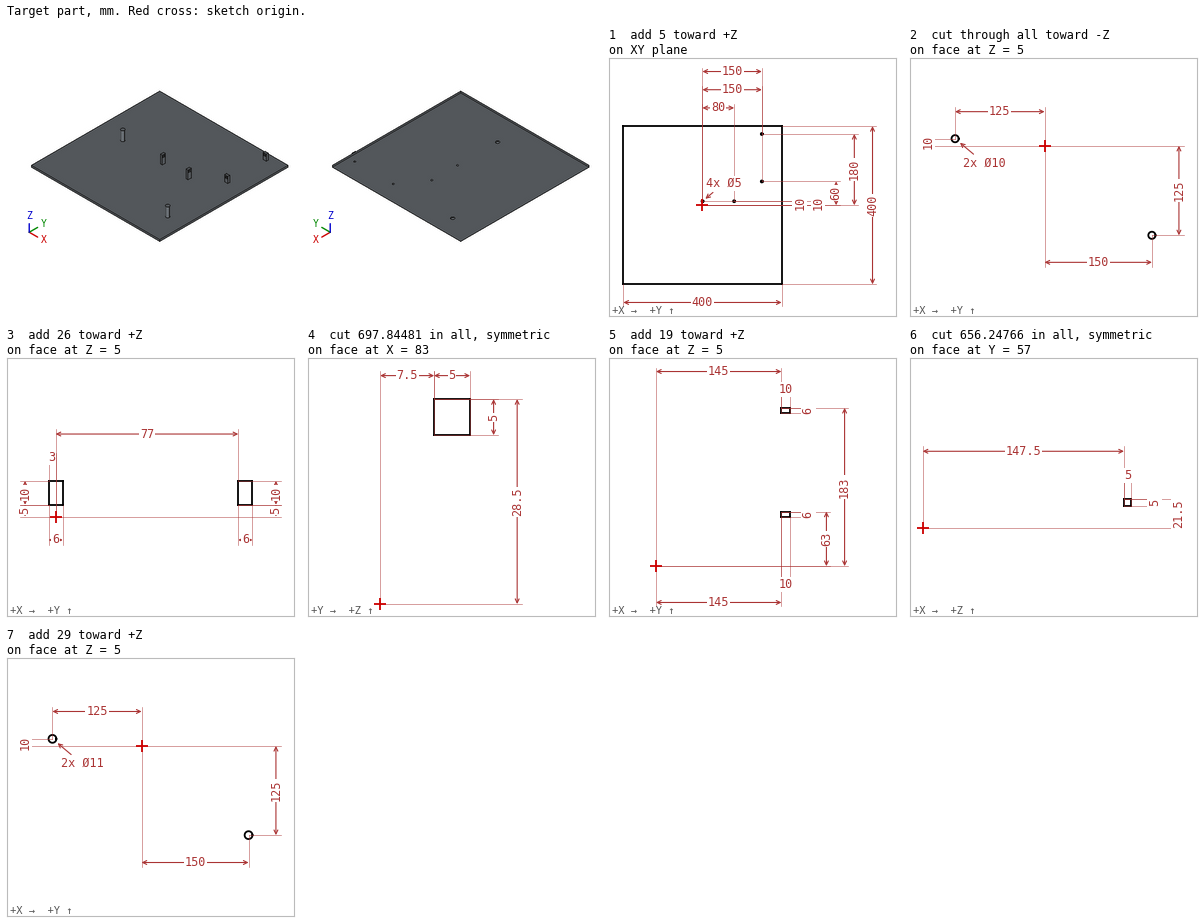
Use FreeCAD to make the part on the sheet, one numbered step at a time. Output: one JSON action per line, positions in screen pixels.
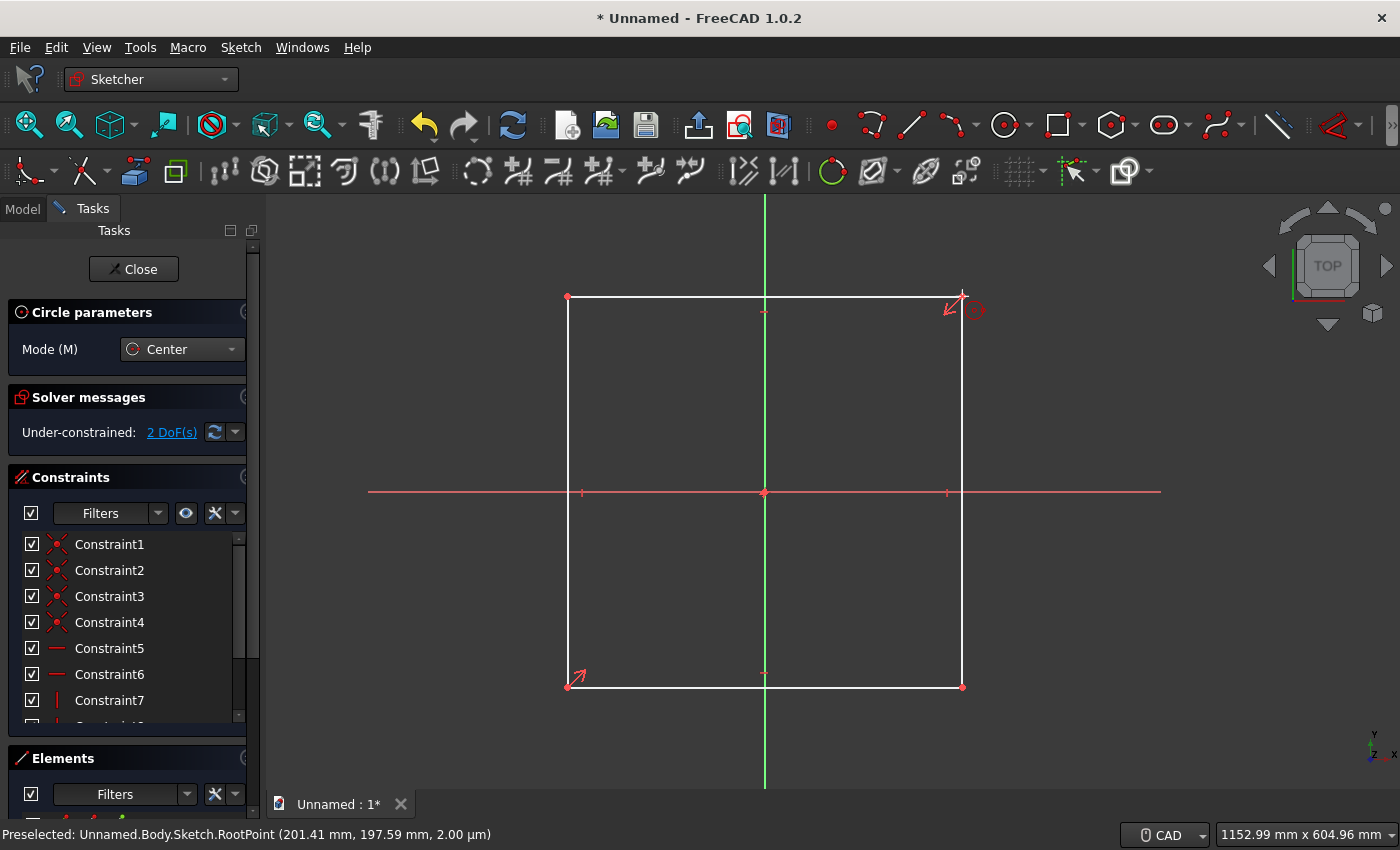
{"action": "scroll", "coordinate": [765, 483], "scroll_direction": "up", "scroll_amount": 12}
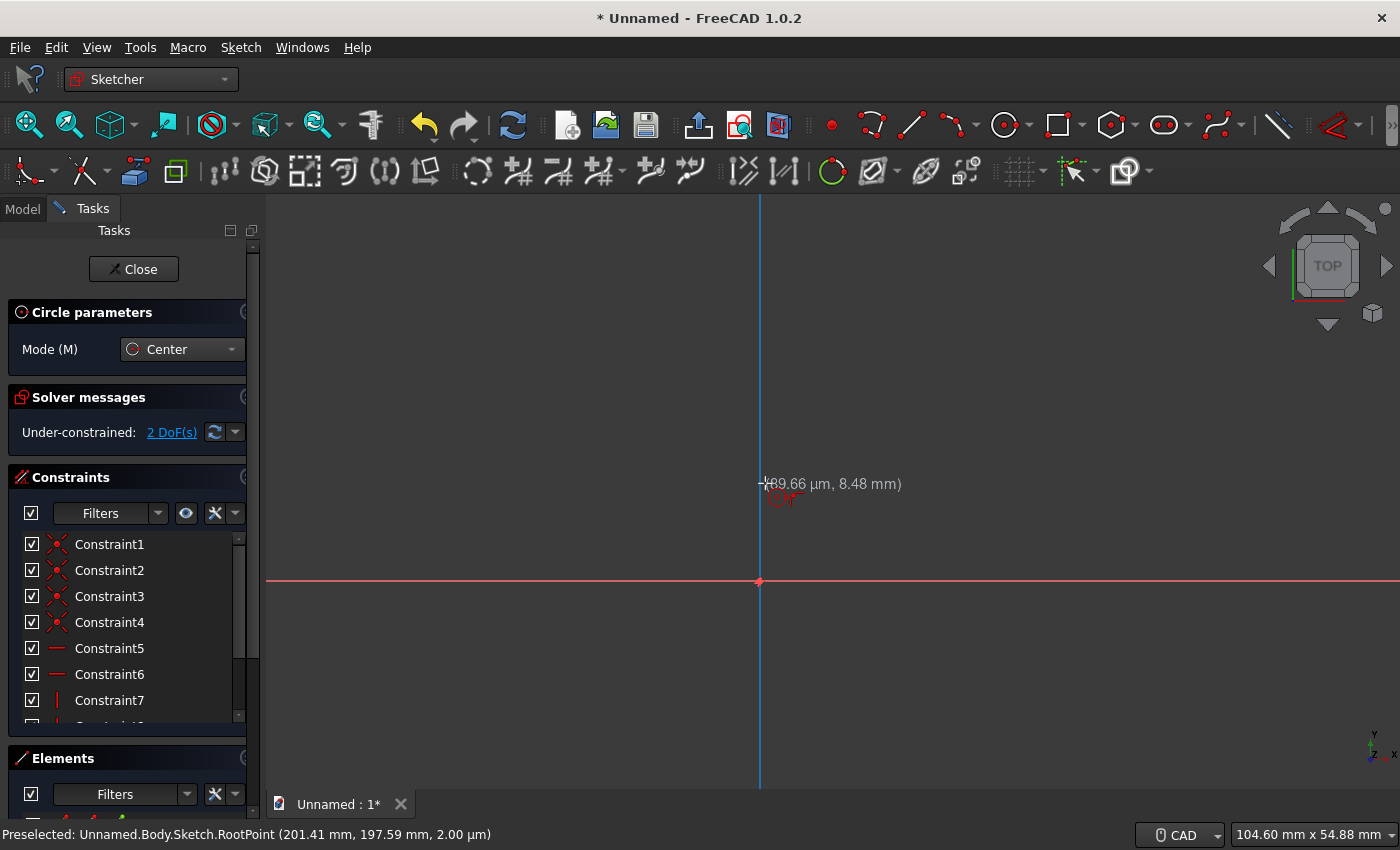
{"action": "scroll", "coordinate": [765, 483], "scroll_direction": "down", "scroll_amount": 12}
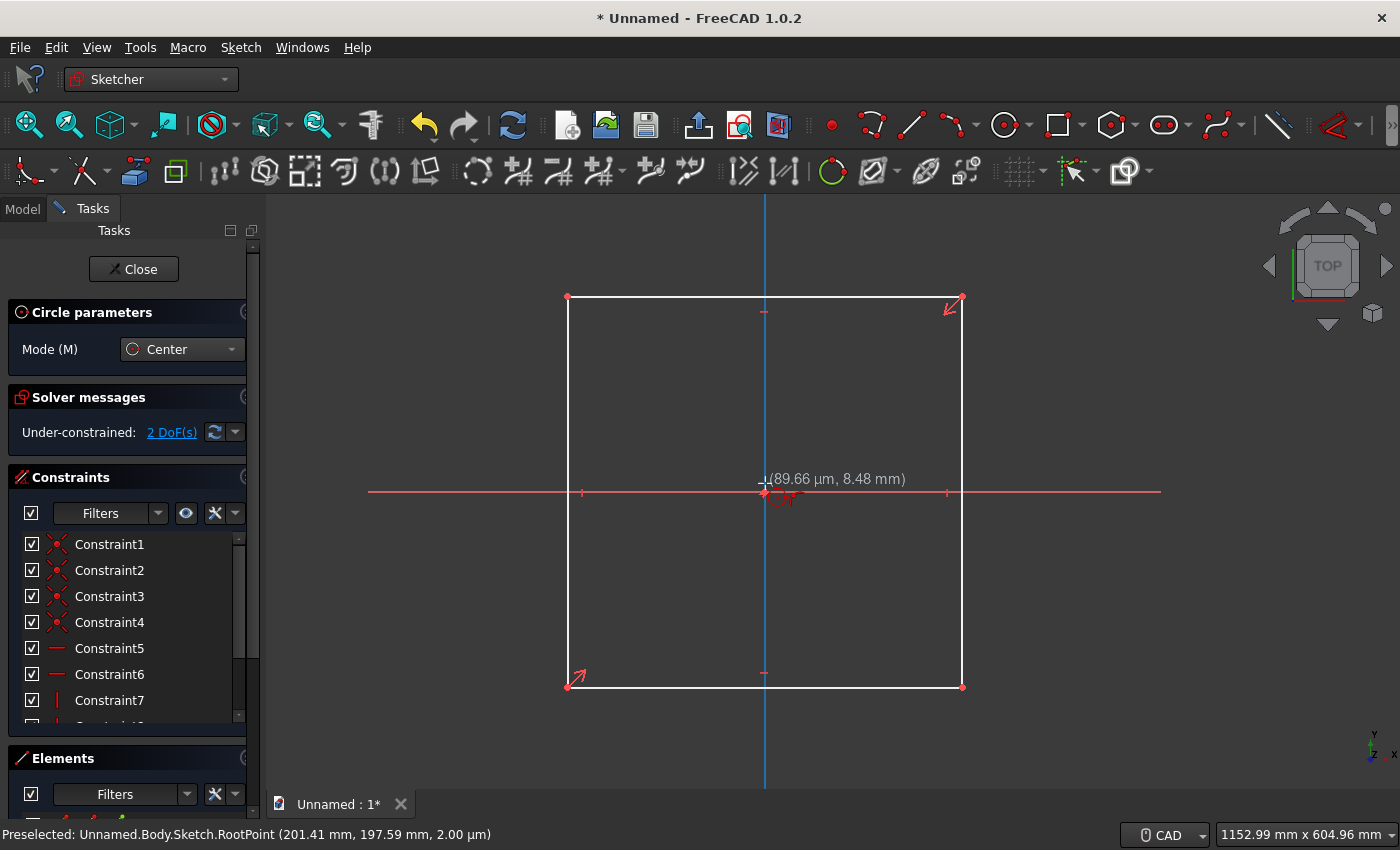
{"action": "scroll", "coordinate": [765, 483], "scroll_direction": "up", "scroll_amount": 3}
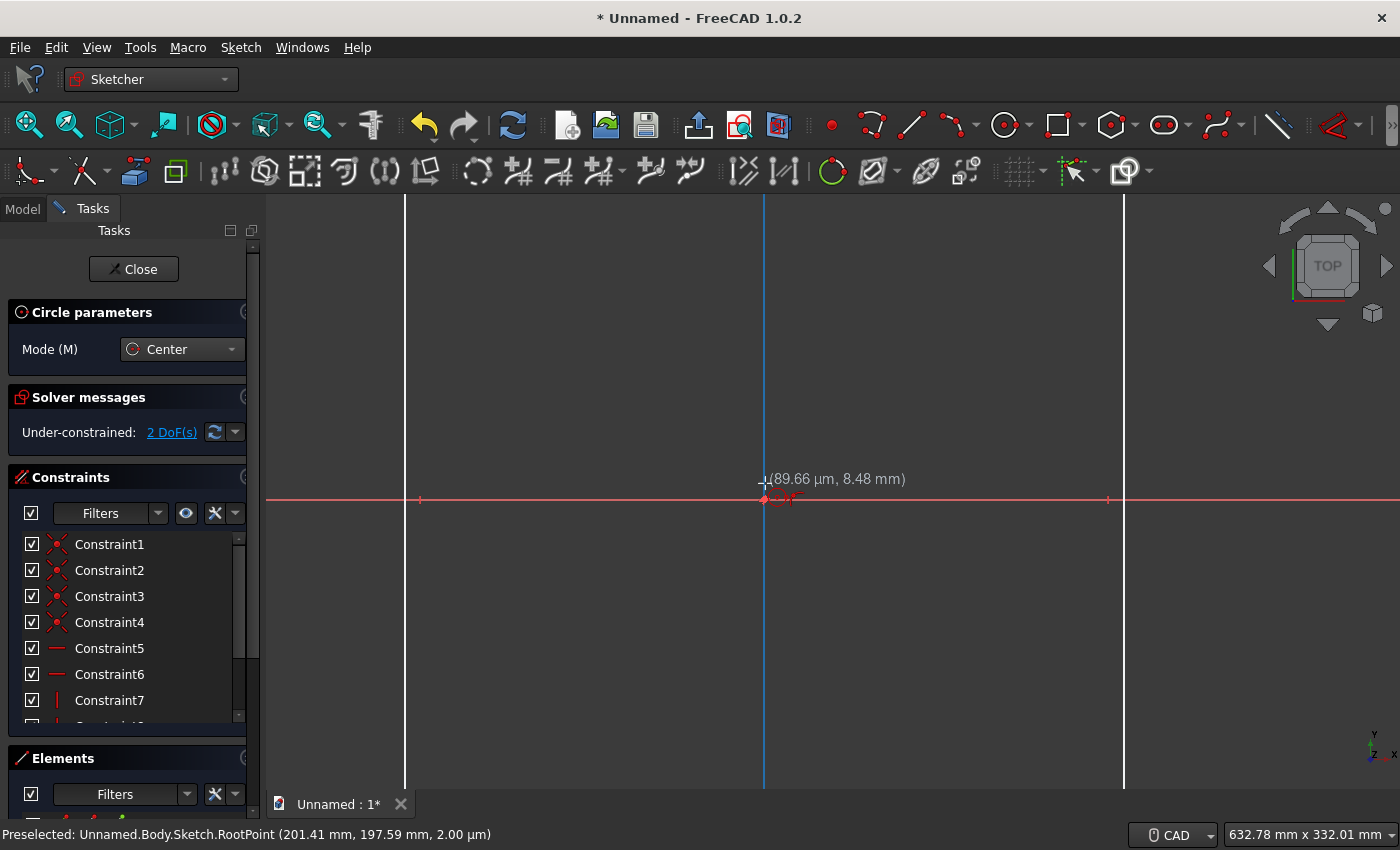
{"action": "left_click", "coordinate": [764, 482]}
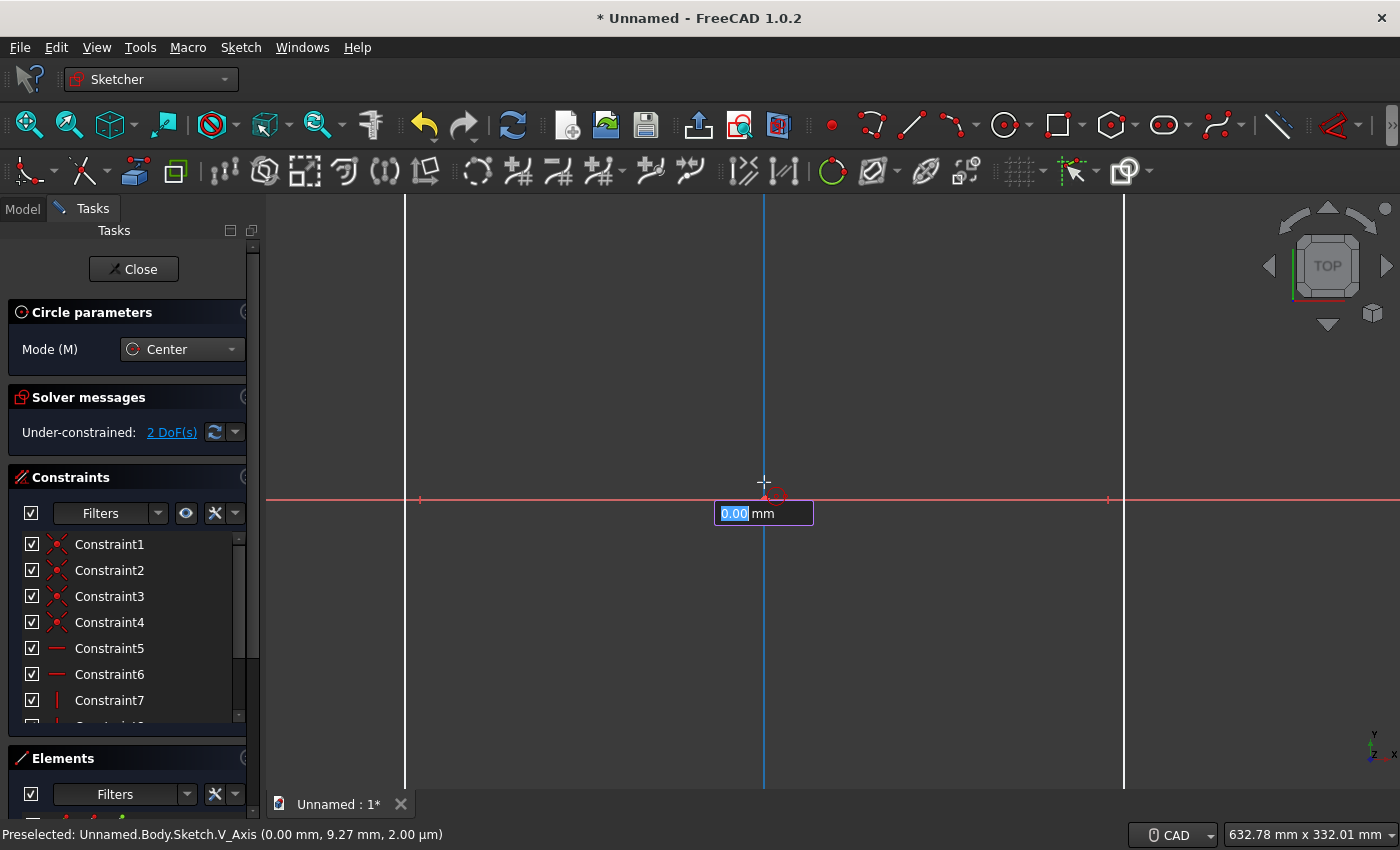
{"action": "scroll", "coordinate": [769, 480], "scroll_direction": "up", "scroll_amount": 7}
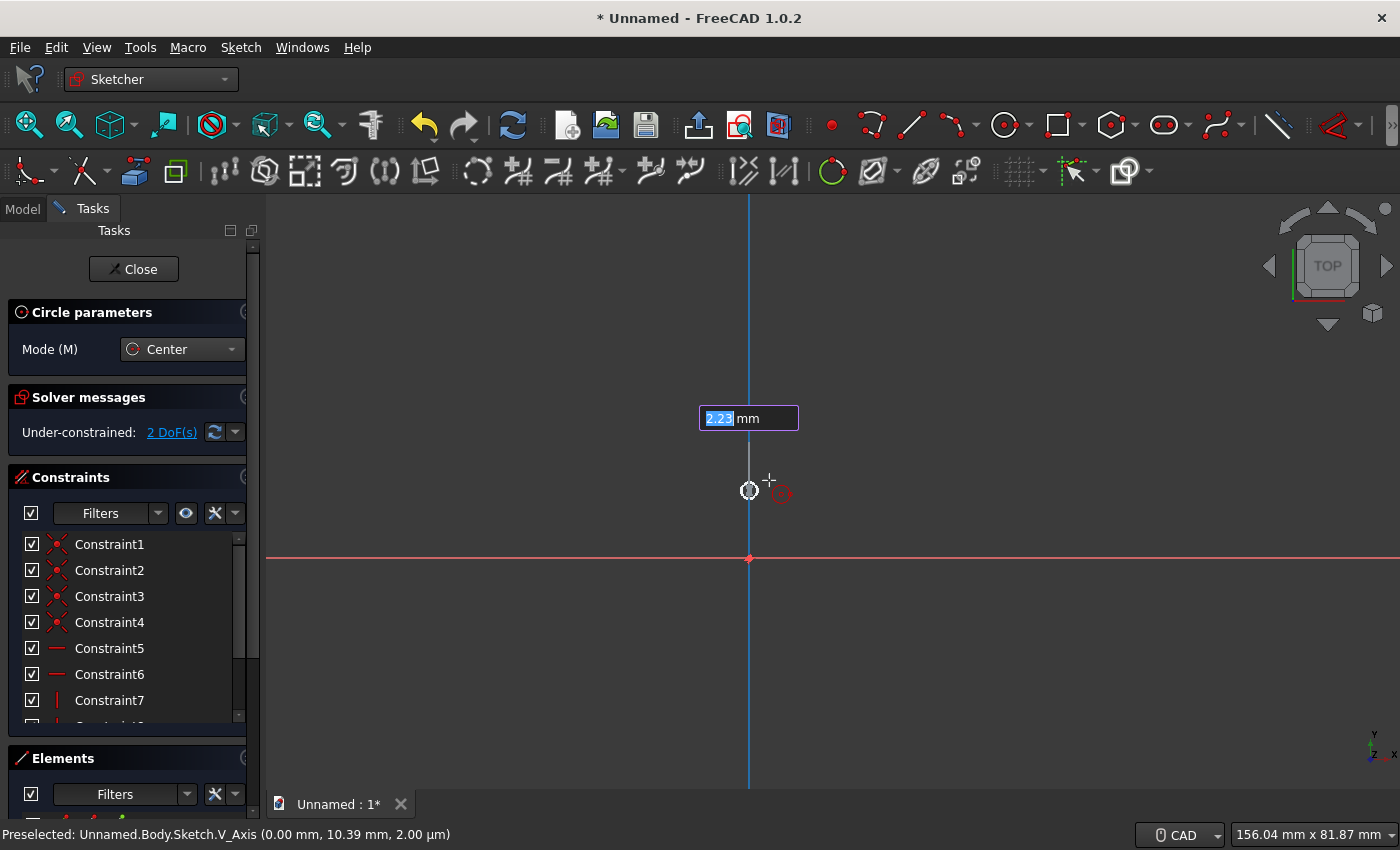
{"action": "left_click", "coordinate": [766, 479]}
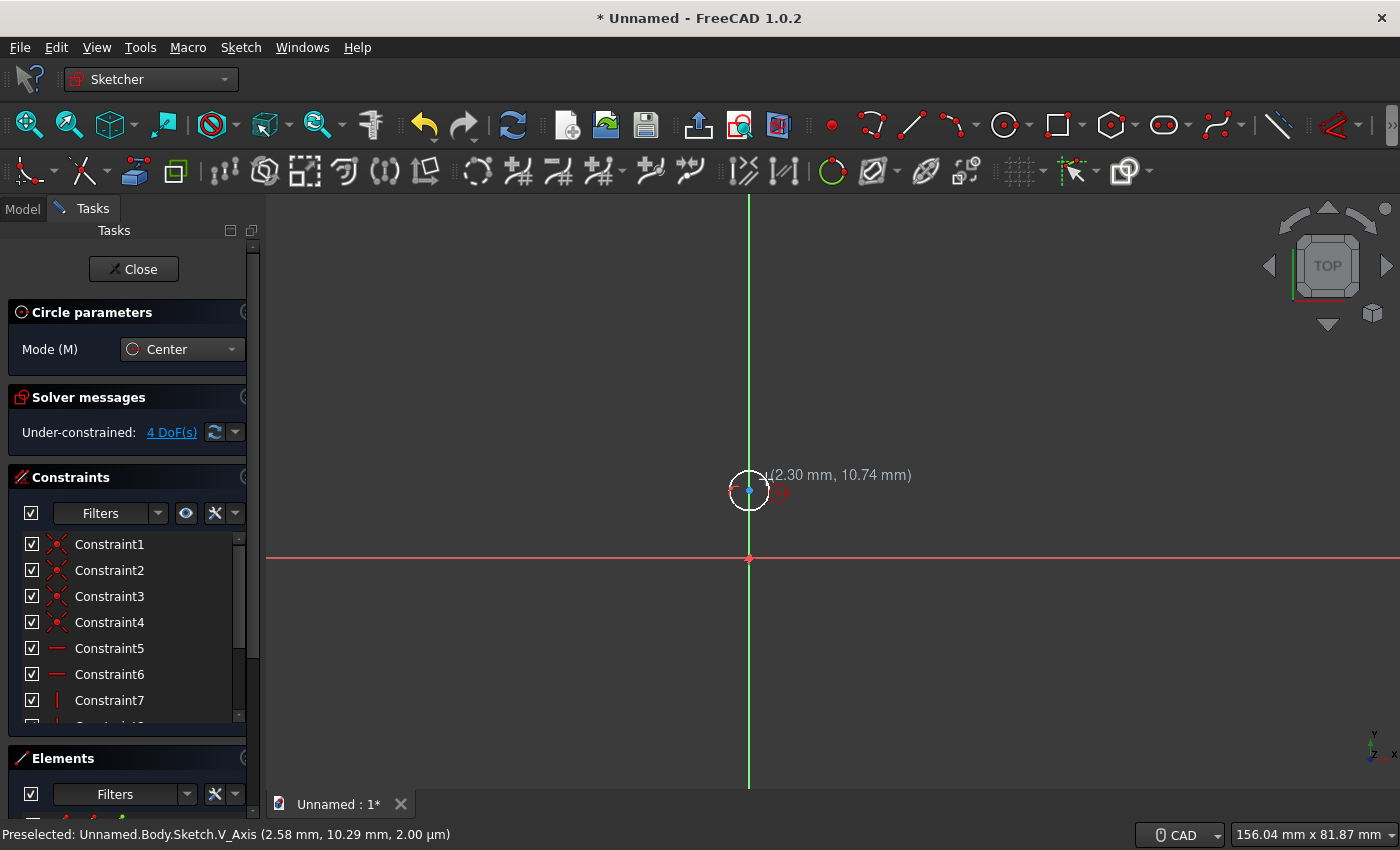
{"action": "scroll", "coordinate": [767, 481], "scroll_direction": "down", "scroll_amount": 10}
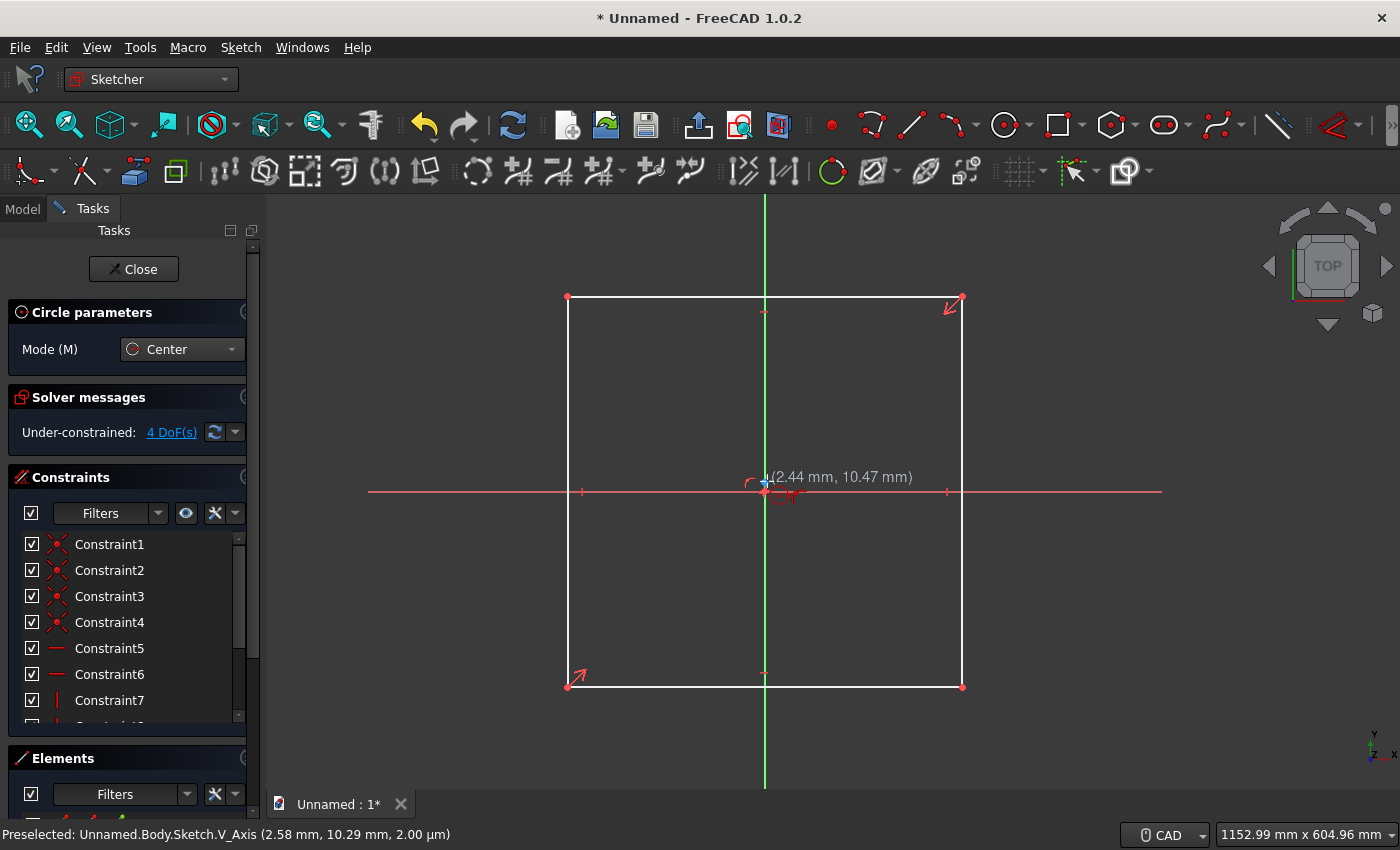
{"action": "scroll", "coordinate": [844, 482], "scroll_direction": "up", "scroll_amount": 12}